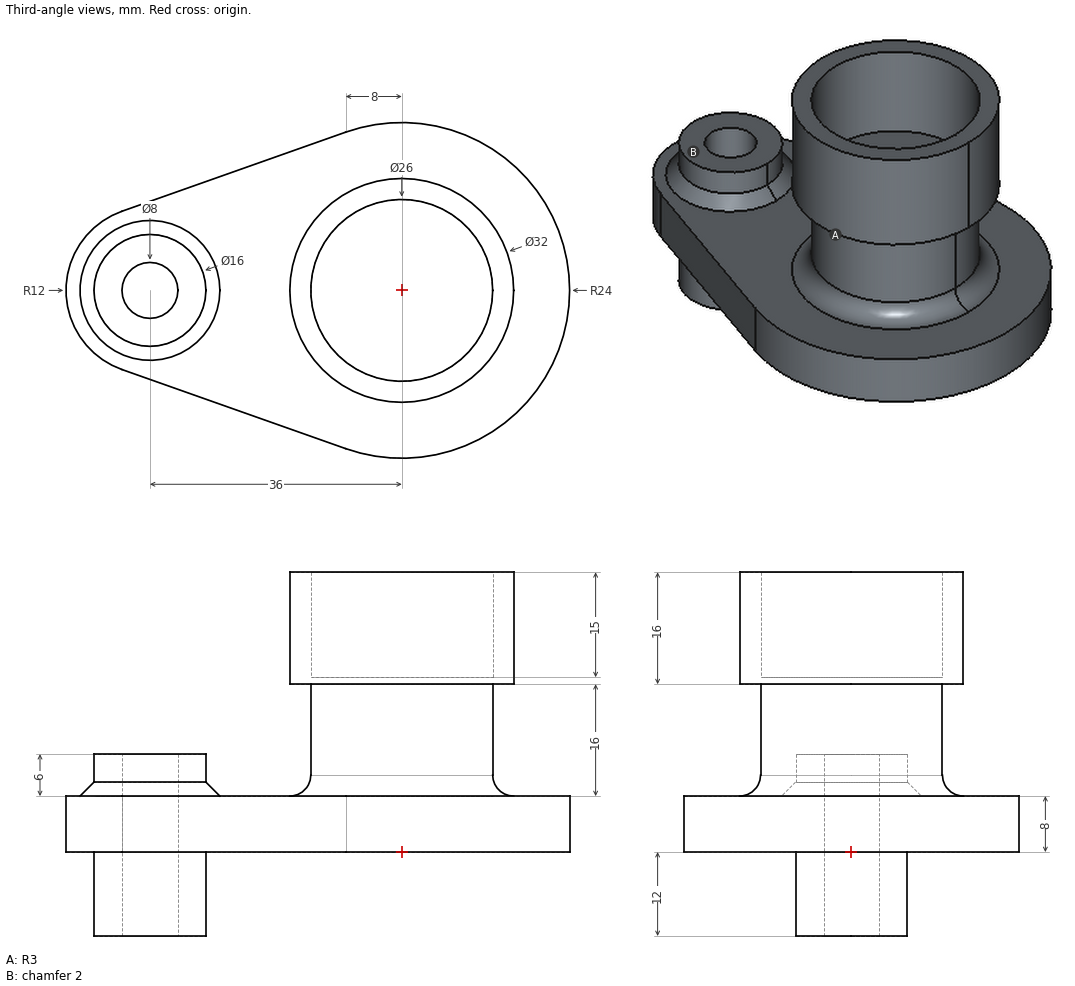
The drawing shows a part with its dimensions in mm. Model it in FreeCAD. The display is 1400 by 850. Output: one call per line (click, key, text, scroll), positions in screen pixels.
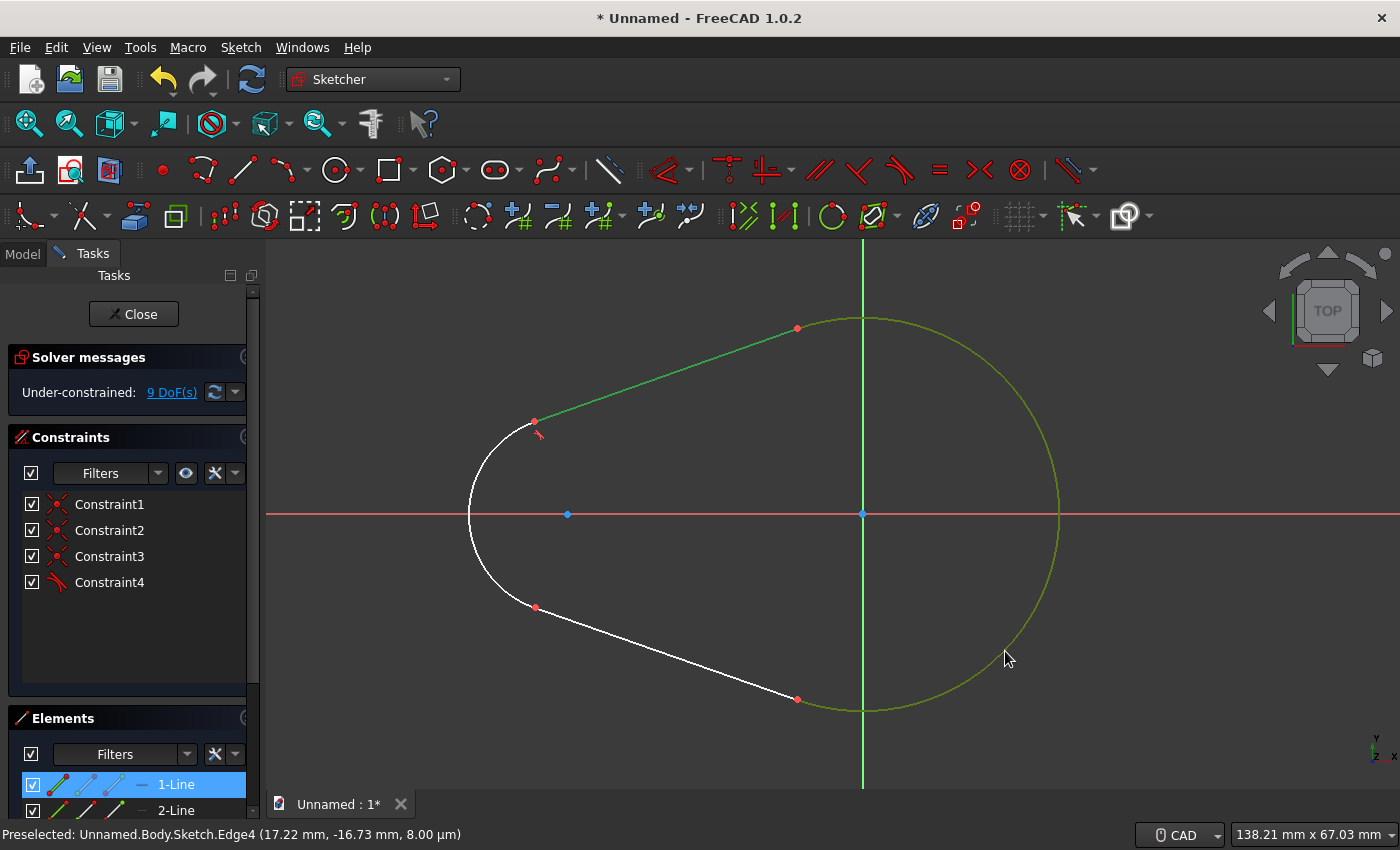
click(900, 170)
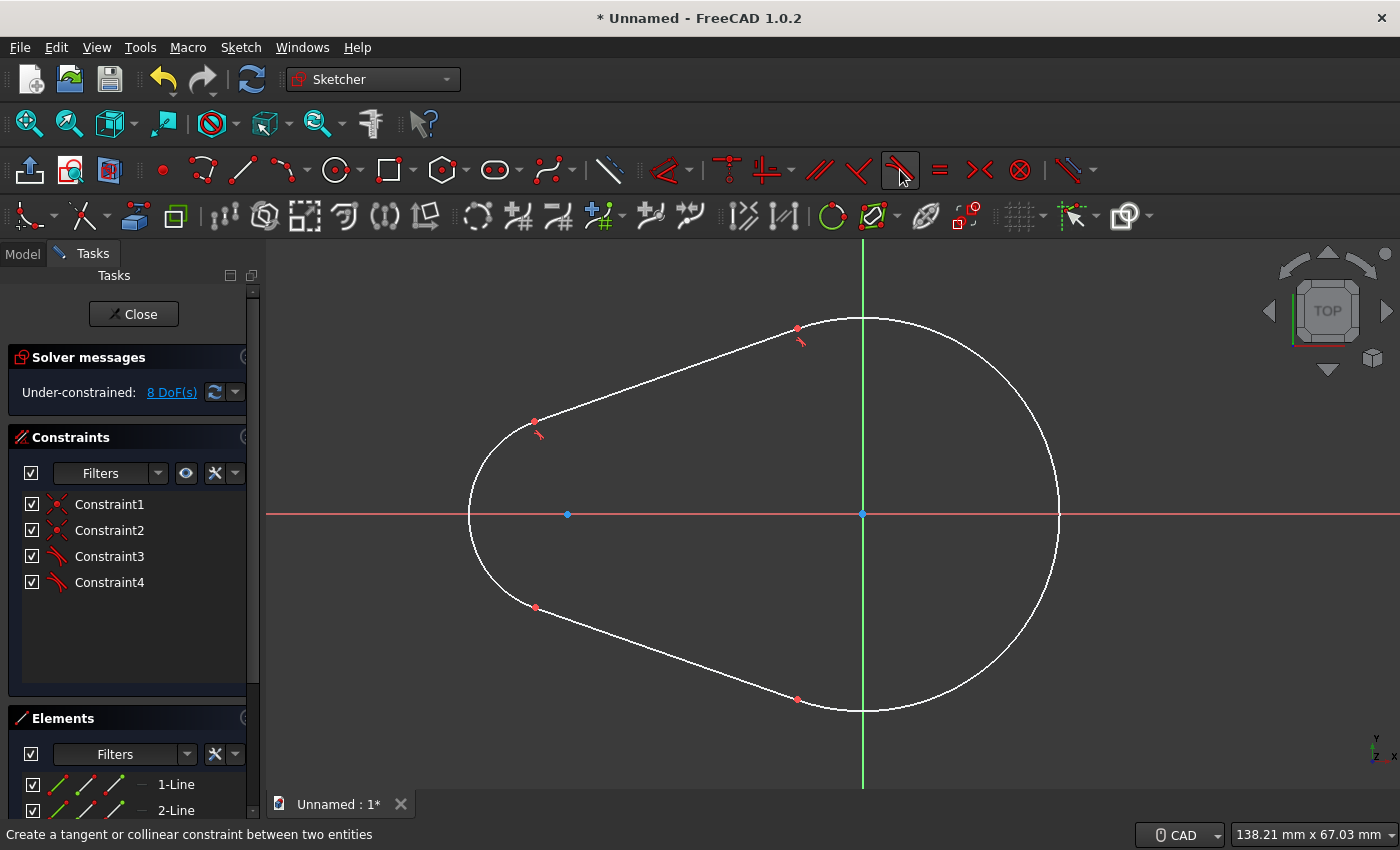
click(614, 636)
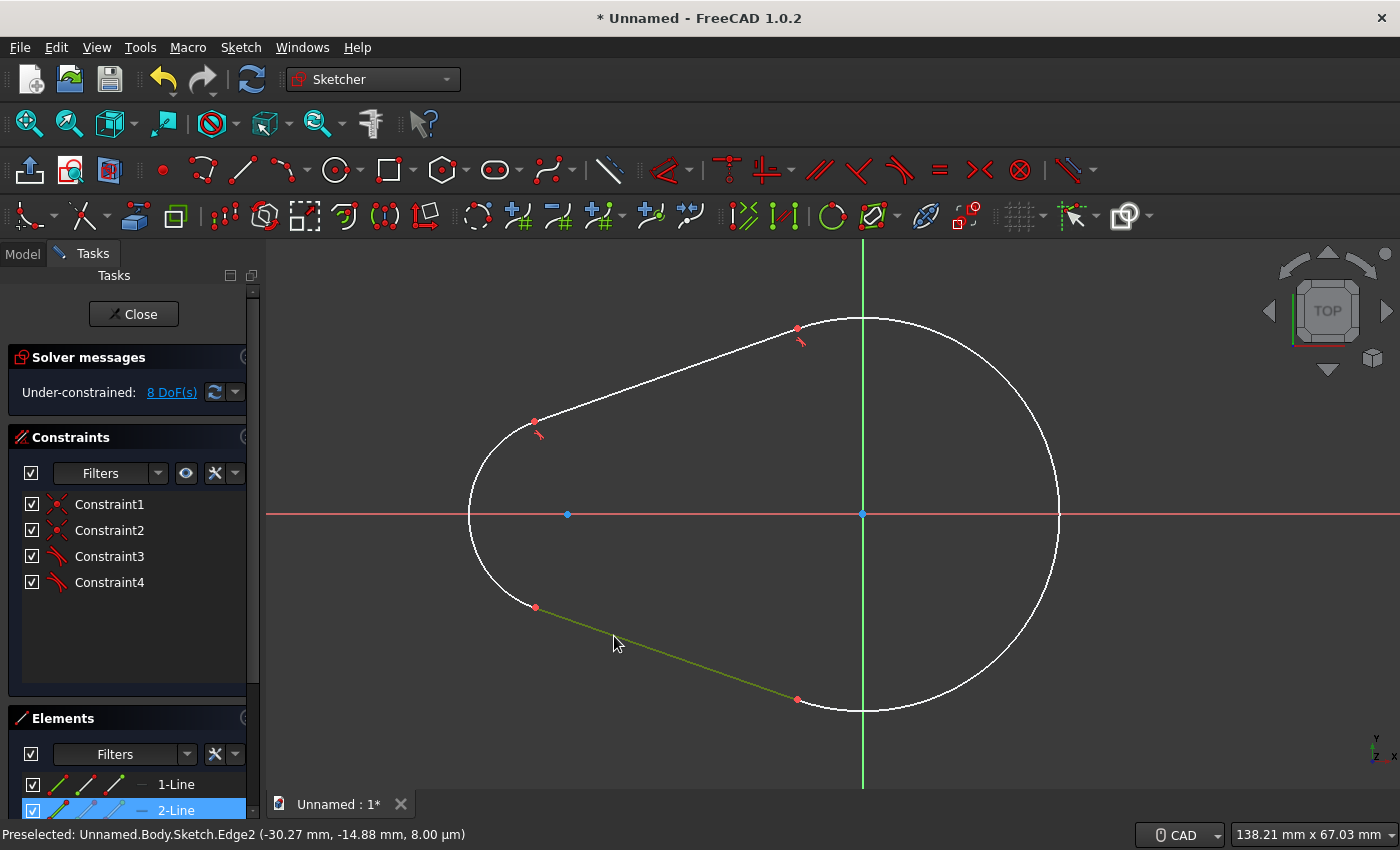
click(481, 468)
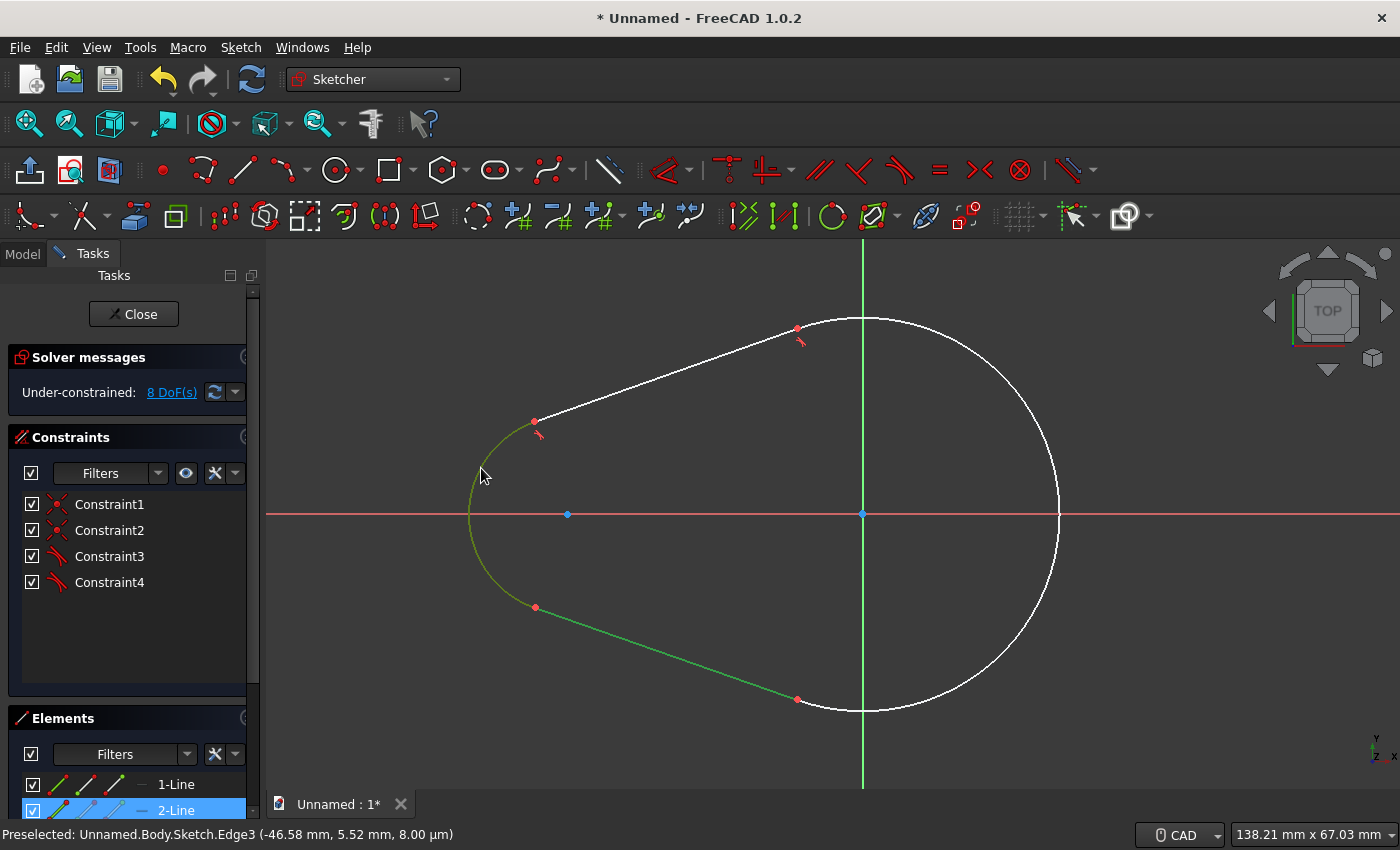
click(900, 170)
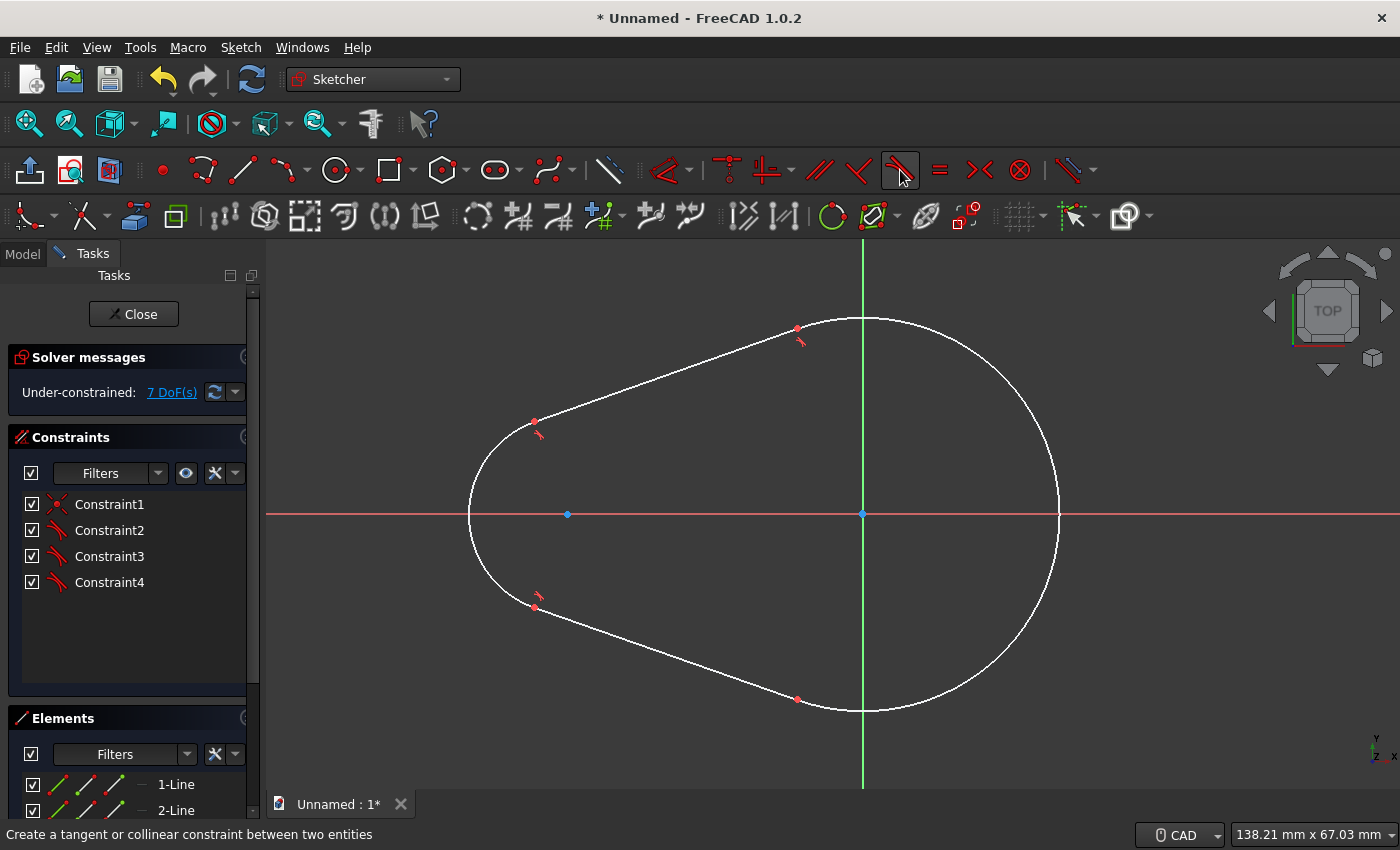
click(614, 636)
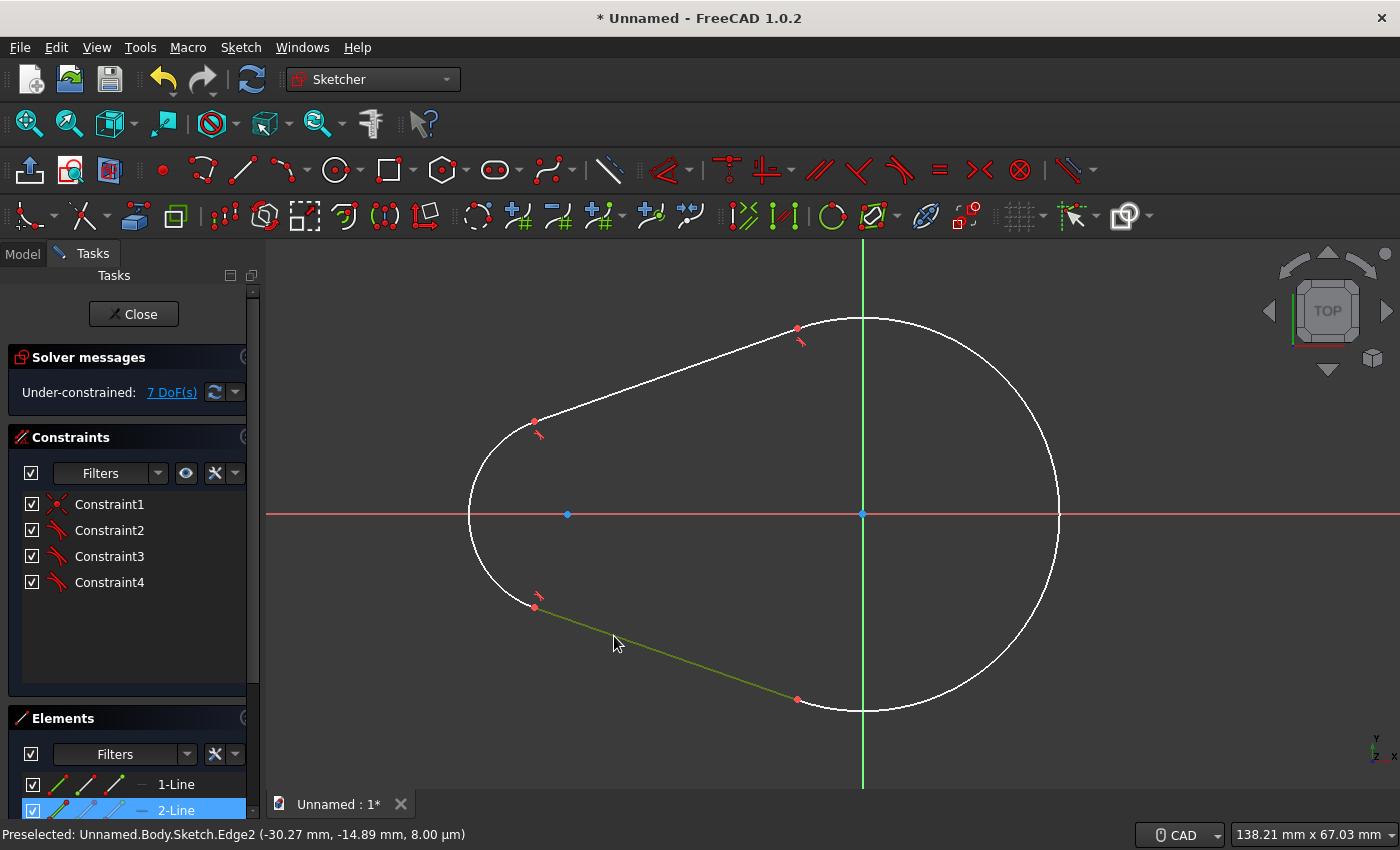
click(1005, 651)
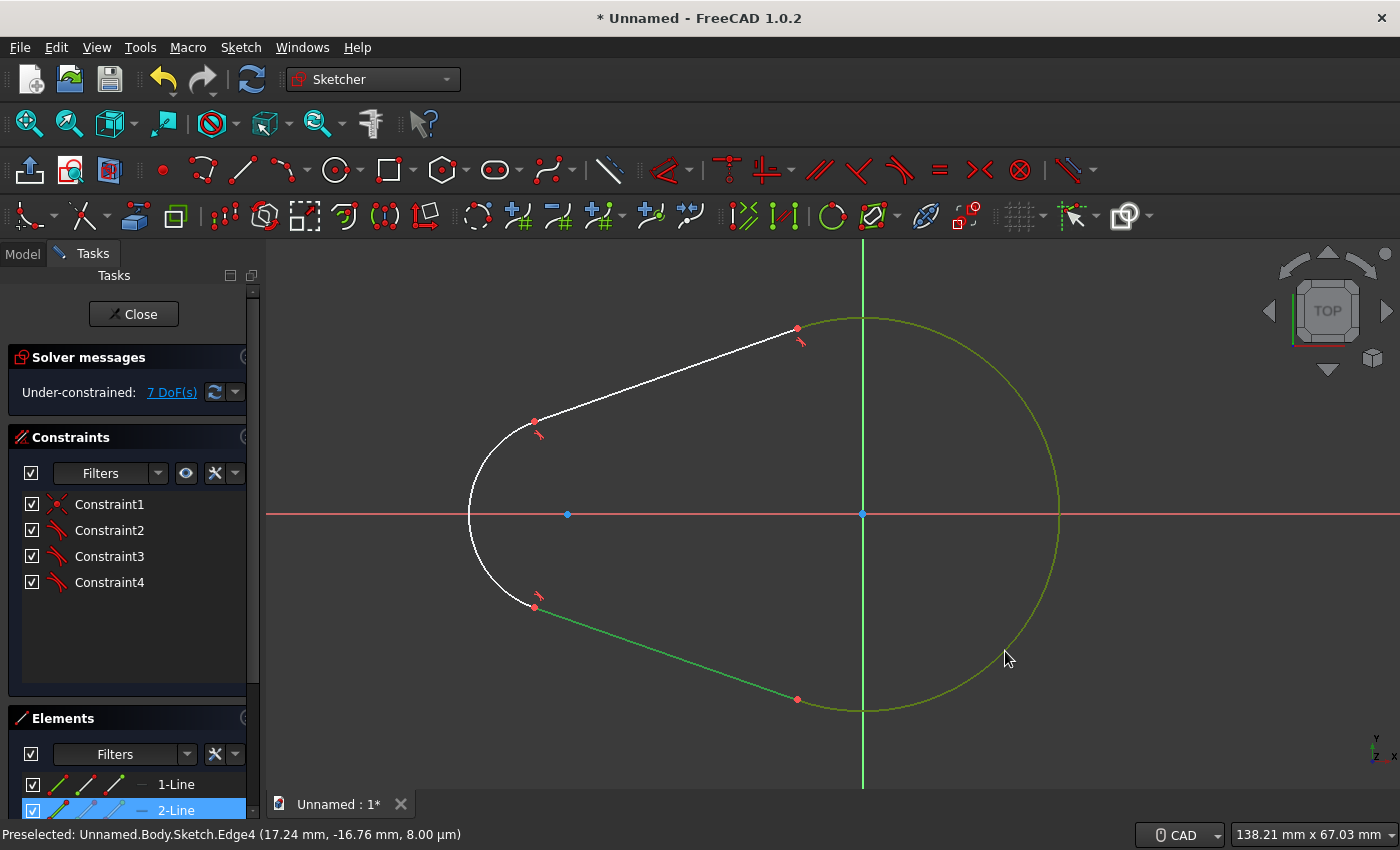
click(900, 170)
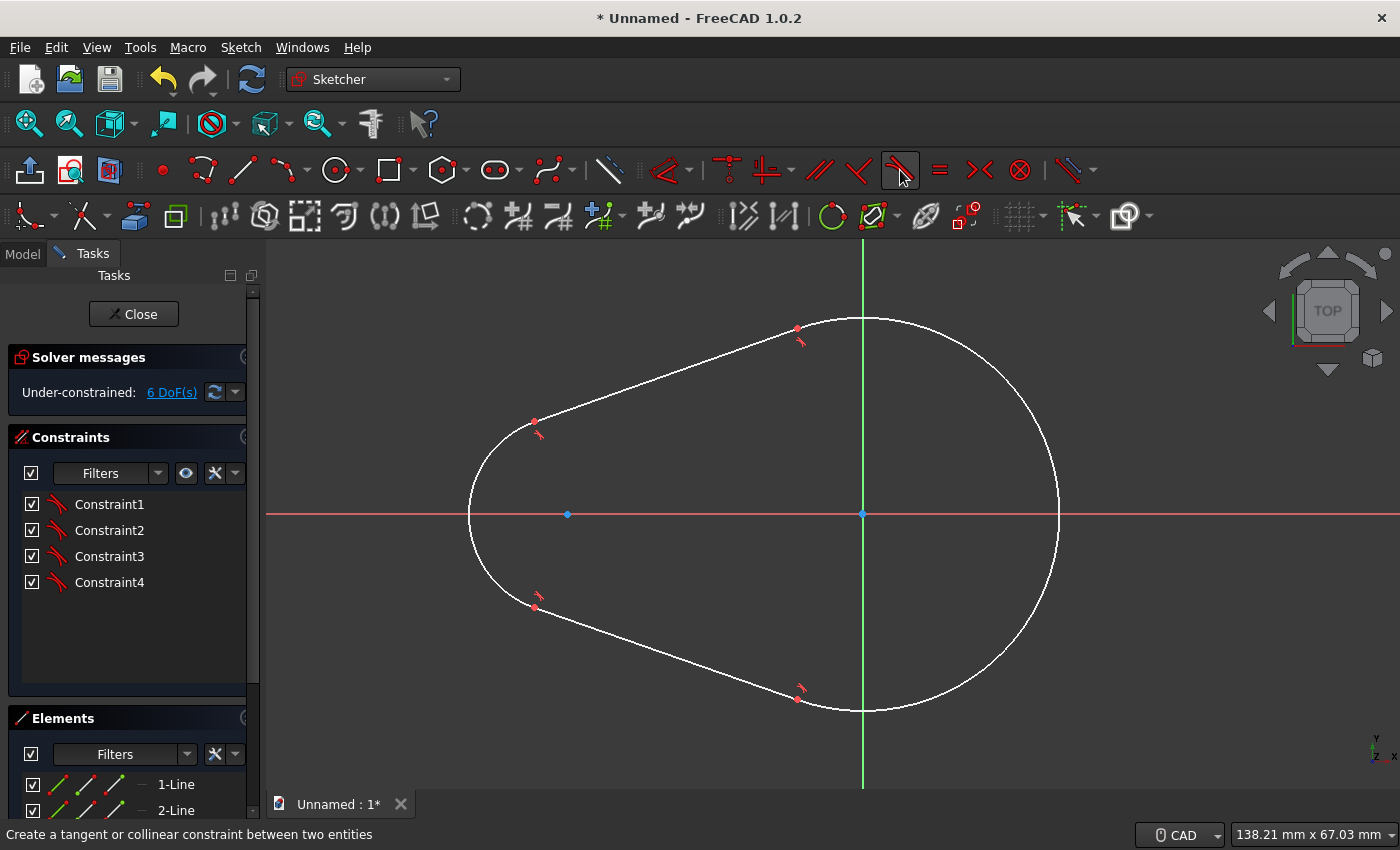
drag(853, 504, 873, 524)